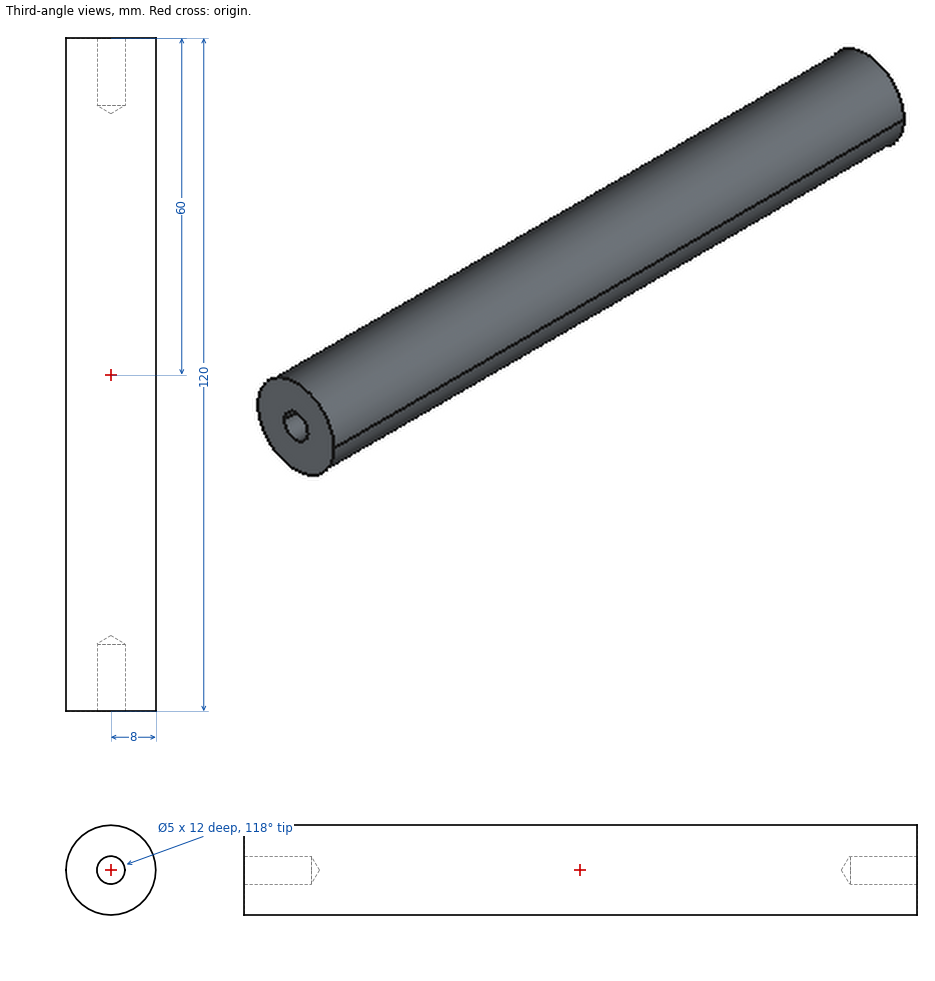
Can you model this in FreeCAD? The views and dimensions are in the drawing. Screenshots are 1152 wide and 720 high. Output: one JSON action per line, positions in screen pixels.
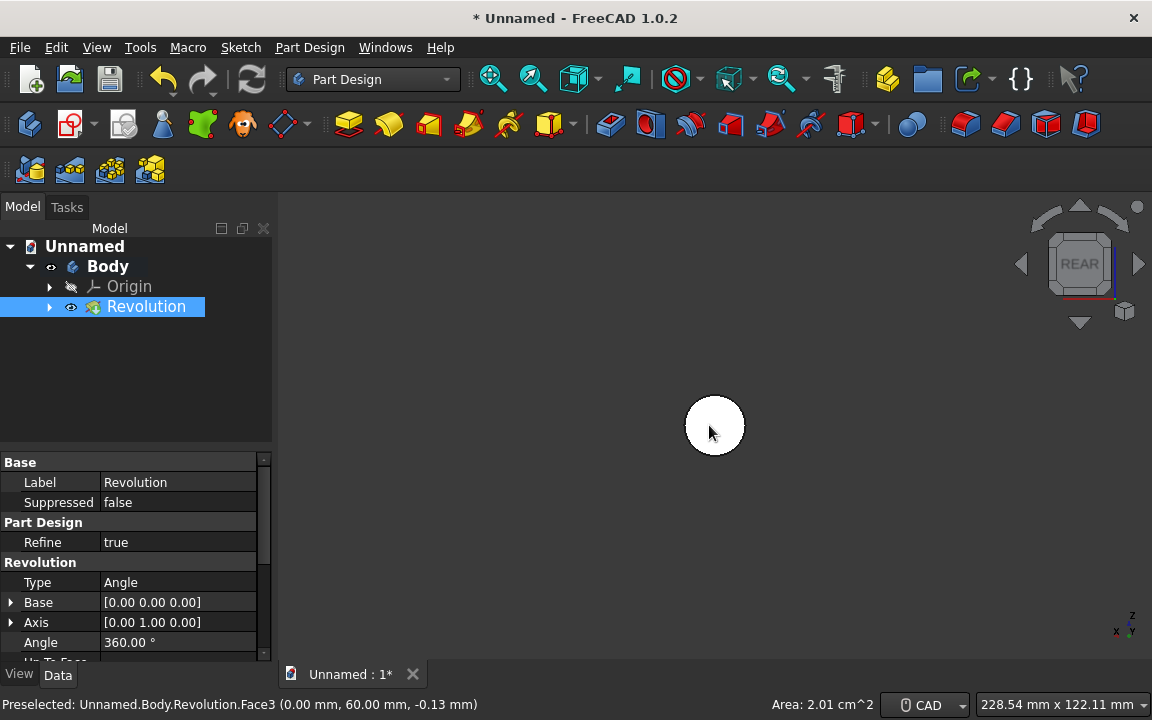
{"action": "left_click", "coordinate": [70, 124]}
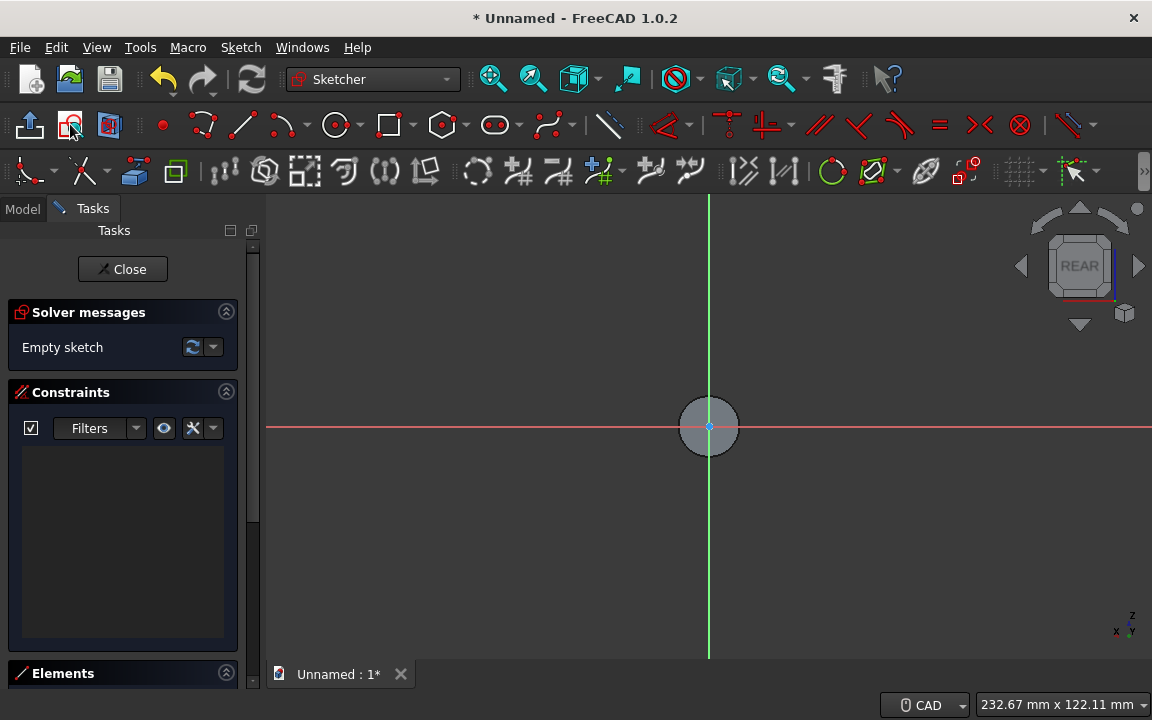
{"action": "scroll", "coordinate": [713, 427], "scroll_direction": "up", "scroll_amount": 14}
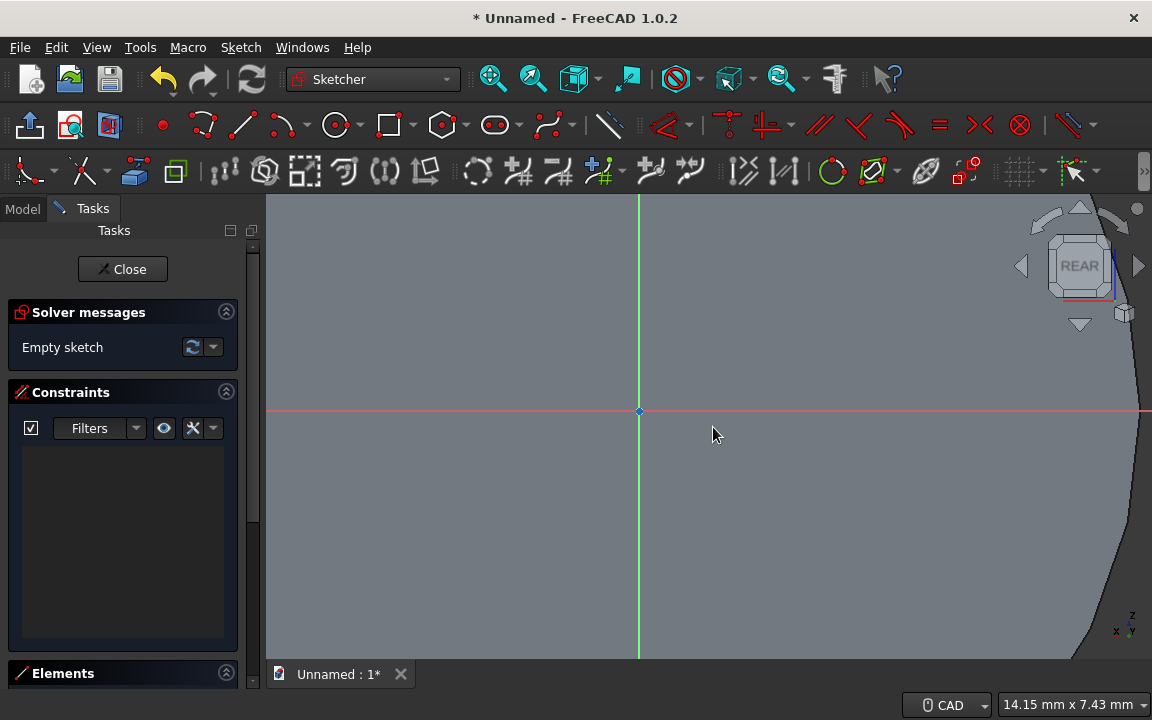
{"action": "key", "text": "g c"}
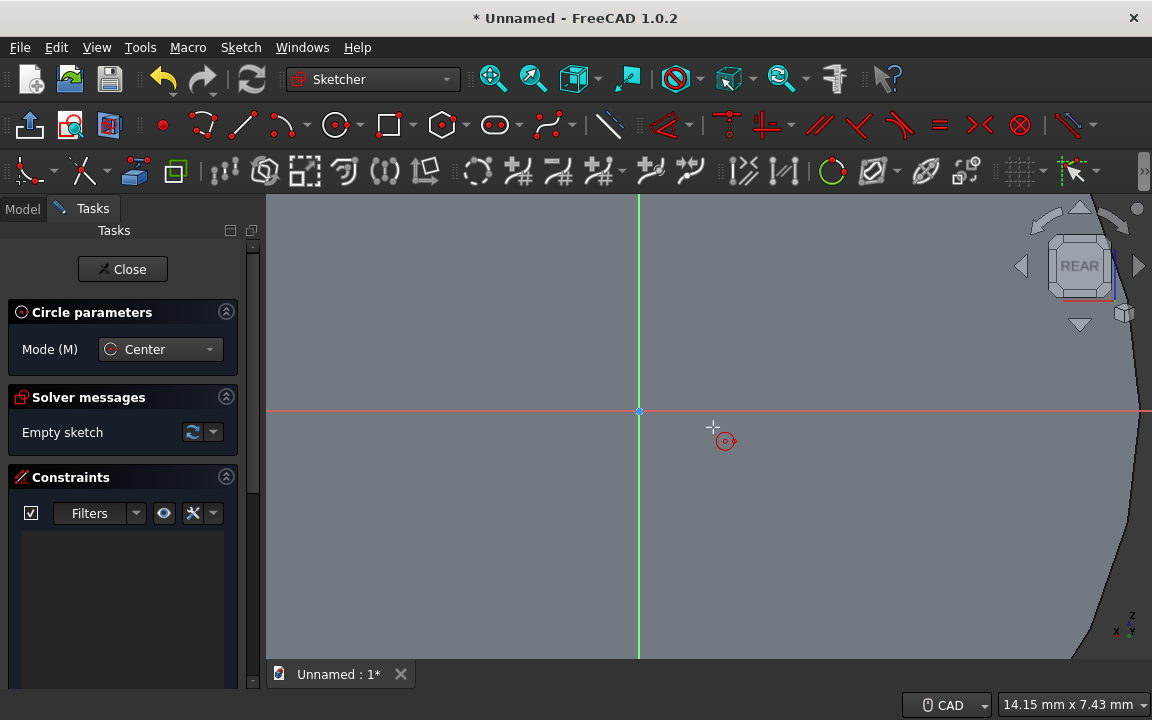
{"action": "left_click", "coordinate": [639, 411]}
{"action": "left_click", "coordinate": [750, 300]}
{"action": "key", "text": "Escape"}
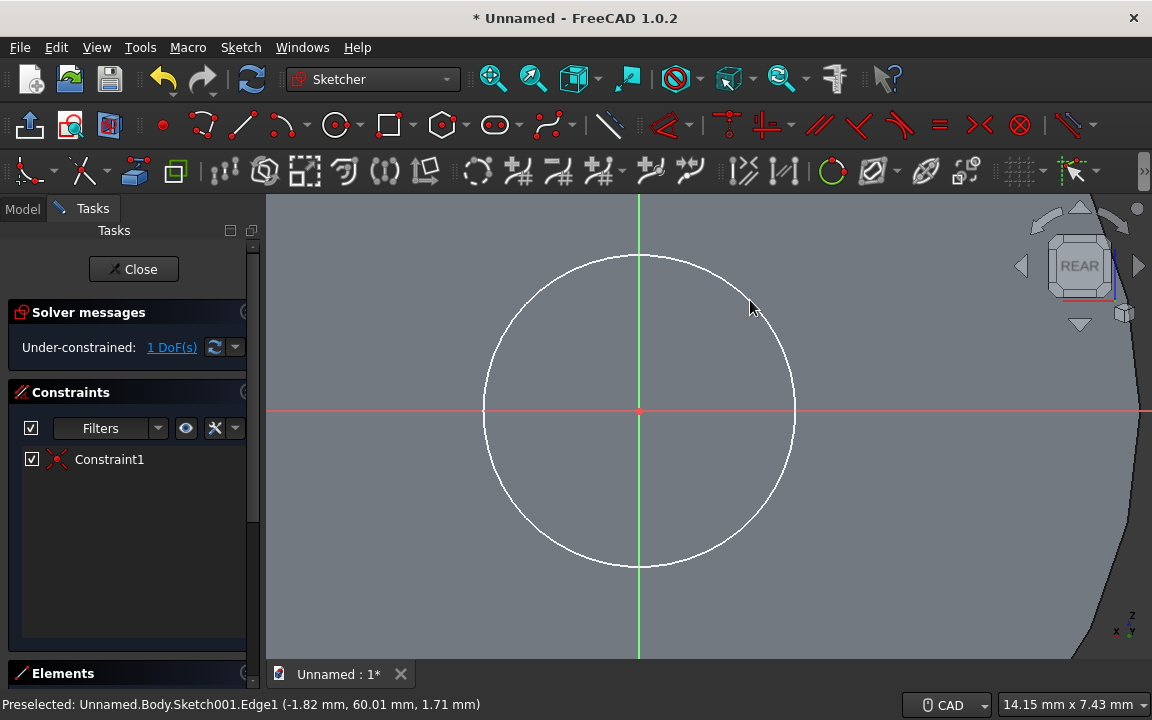
{"action": "left_click", "coordinate": [749, 300]}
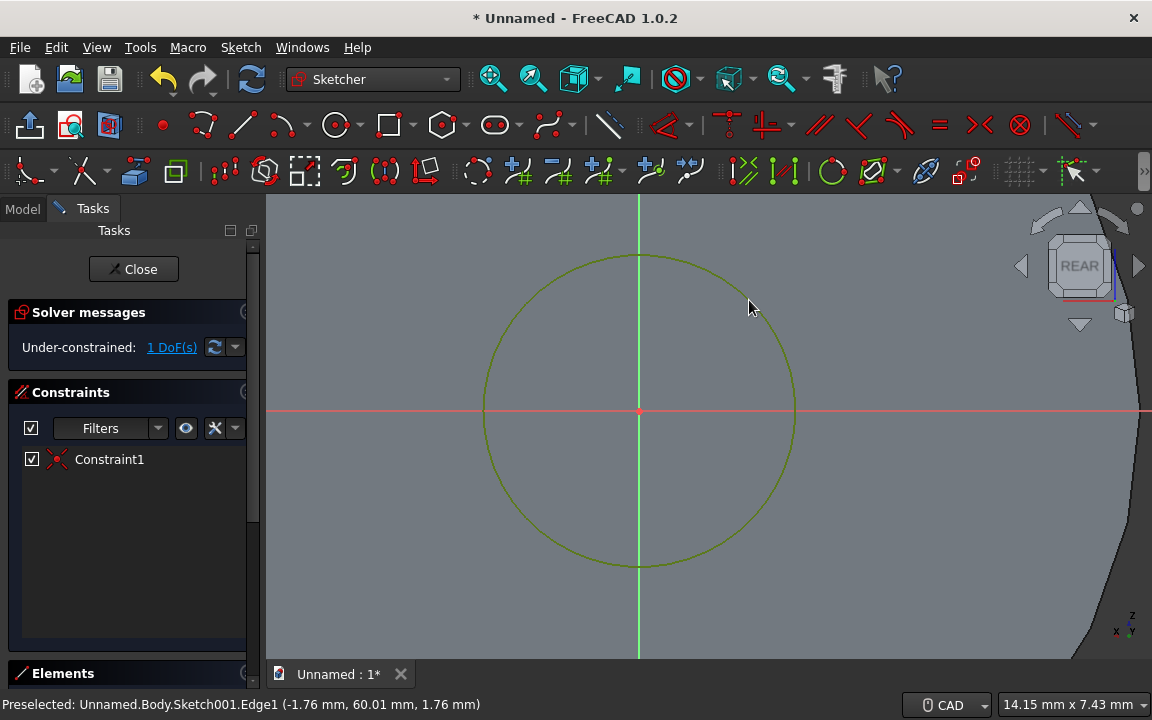
{"action": "key", "text": "k o"}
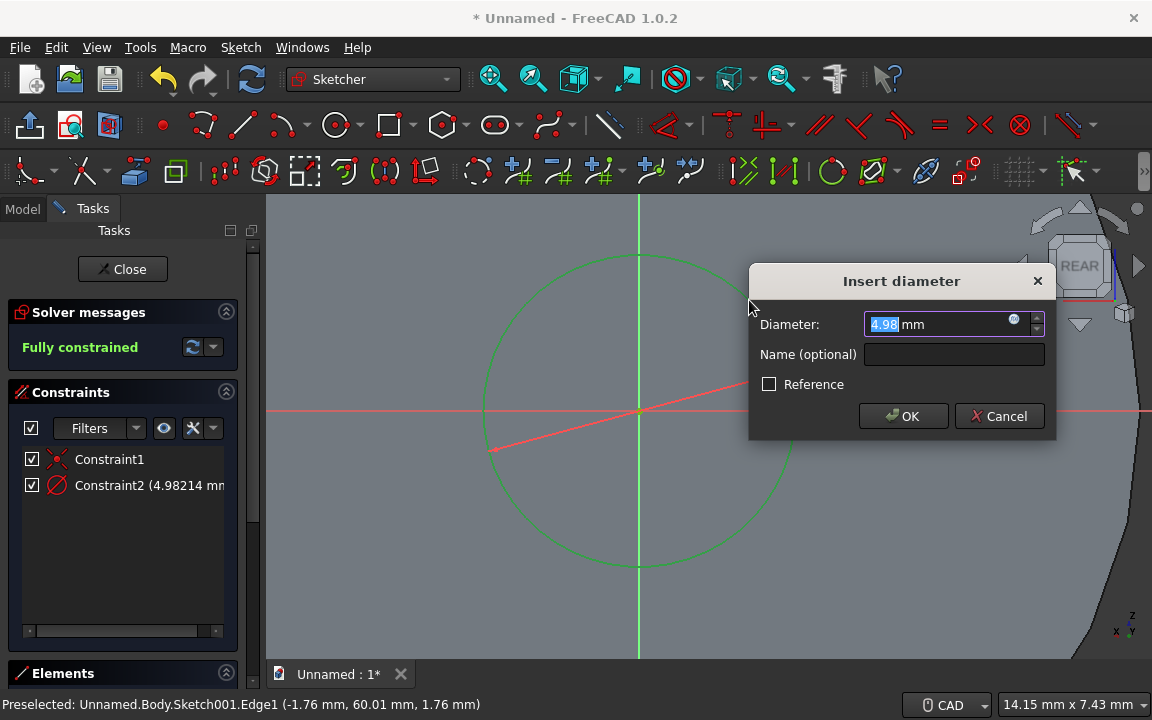
{"action": "type", "text": "5"}
{"action": "key", "text": "Return"}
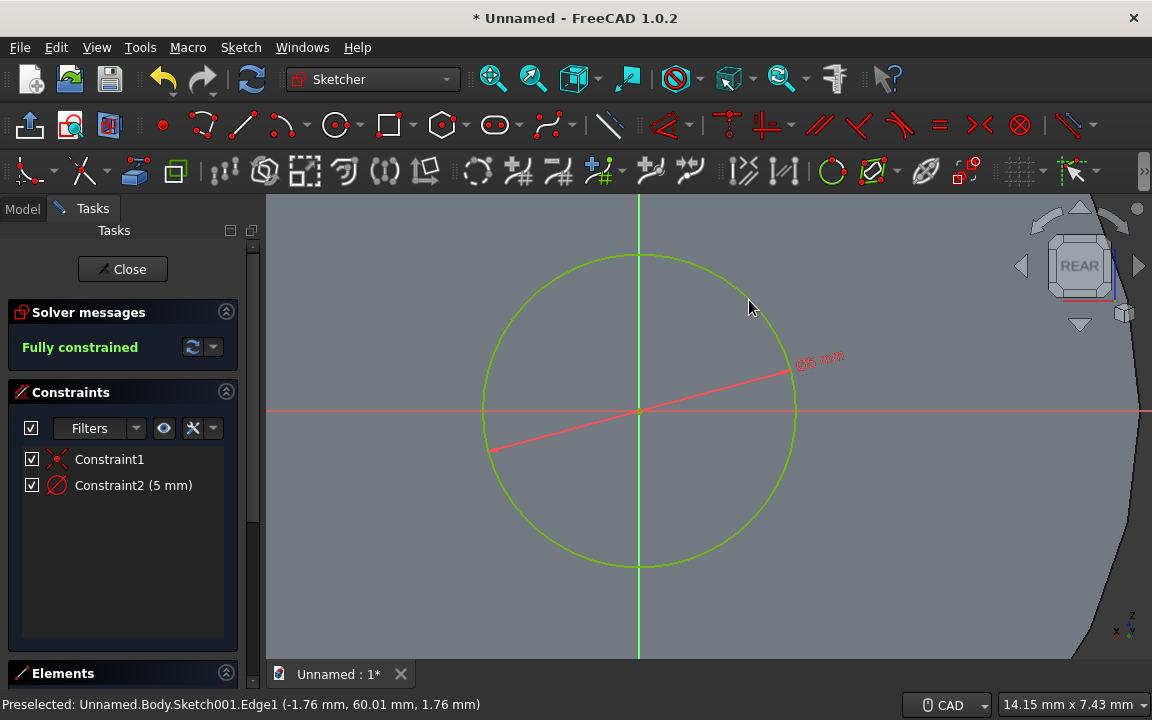
{"action": "left_click", "coordinate": [123, 269]}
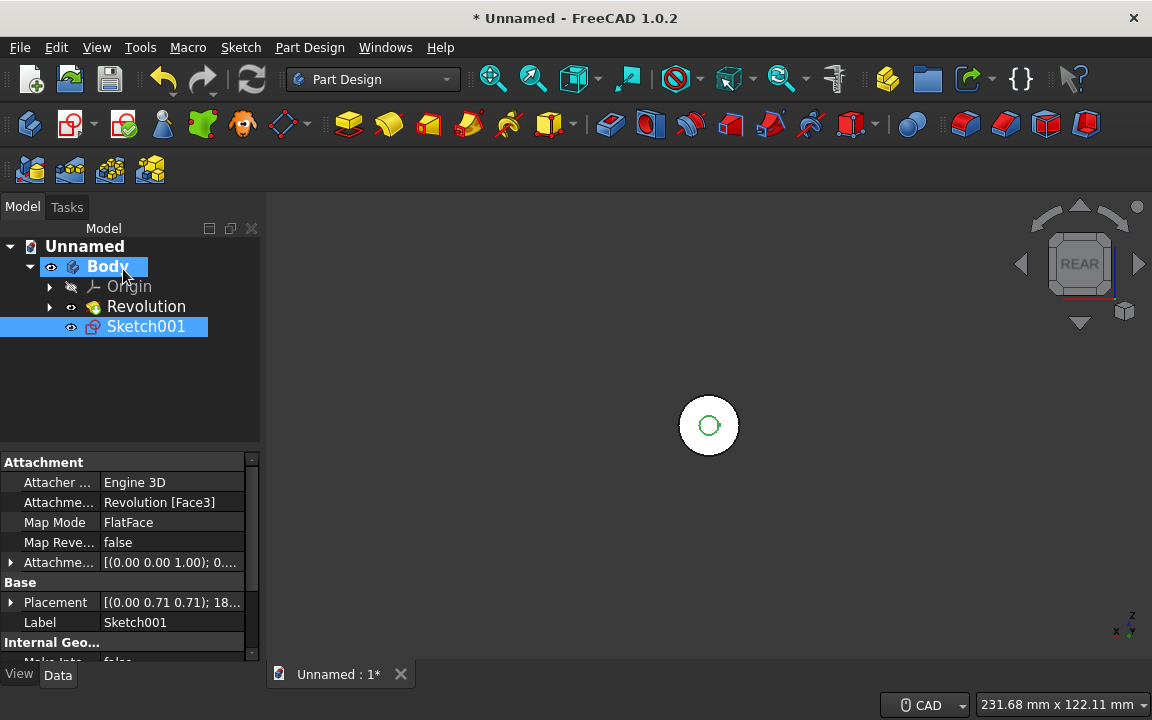
{"action": "left_click", "coordinate": [652, 124]}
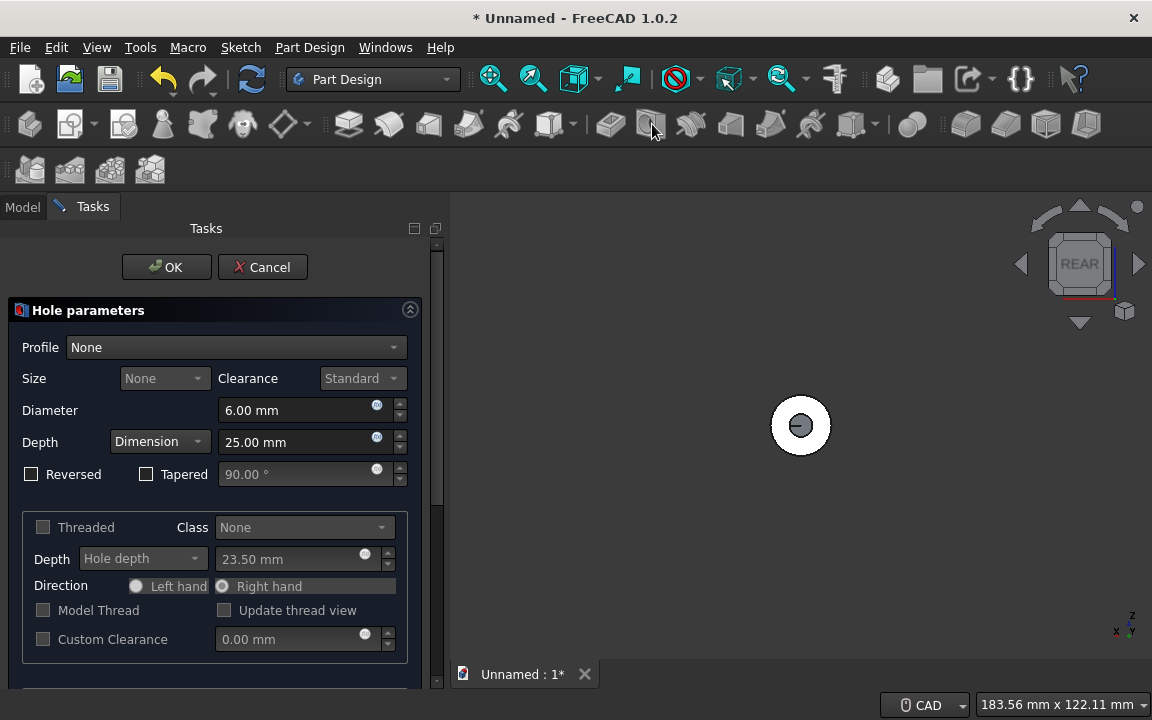
{"action": "triple_click", "coordinate": [305, 410]}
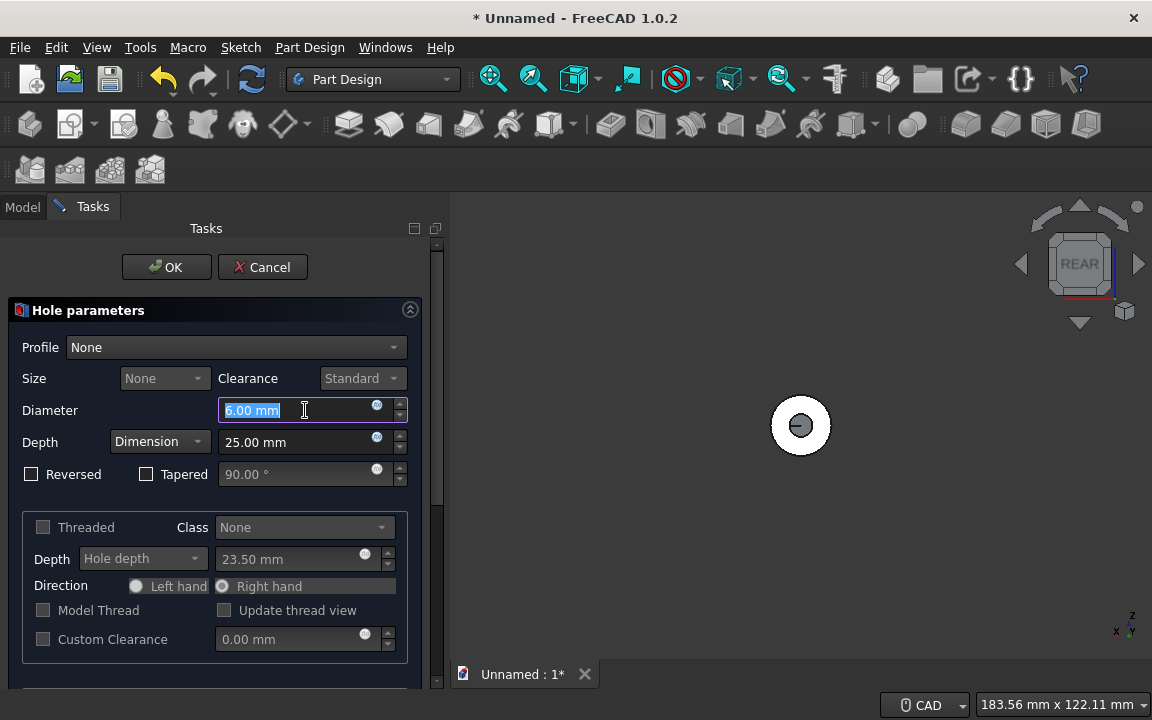
{"action": "type", "text": "5"}
{"action": "key", "text": "Tab"}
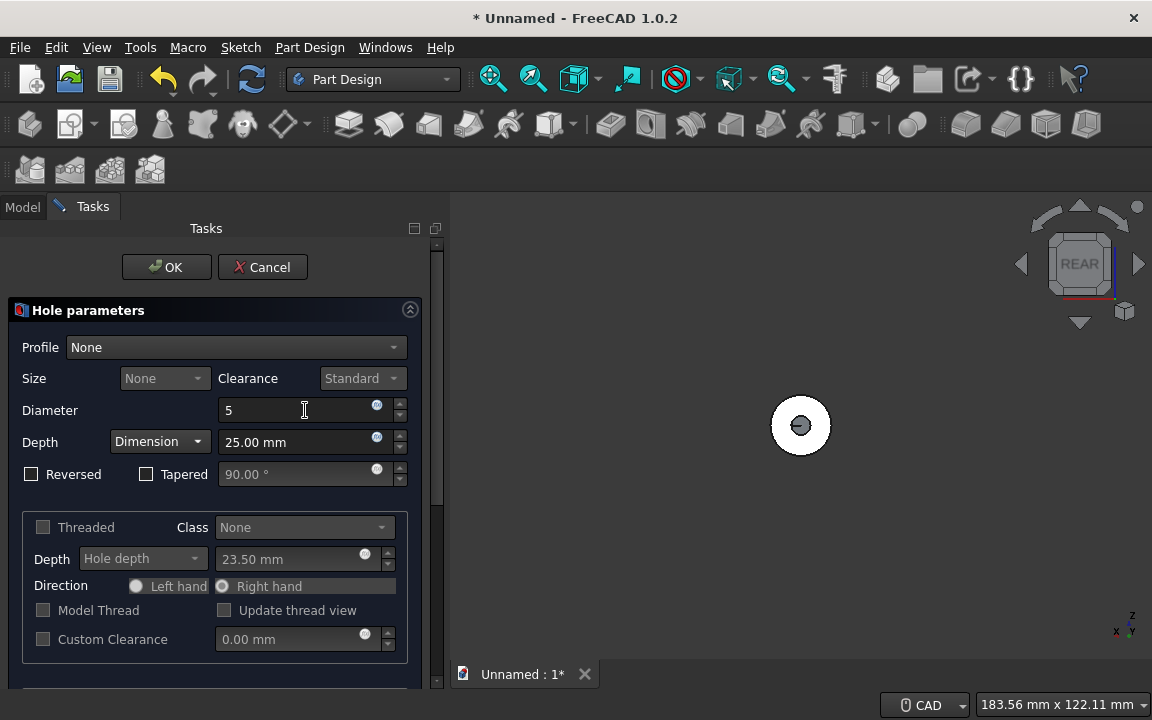
{"action": "triple_click", "coordinate": [305, 442]}